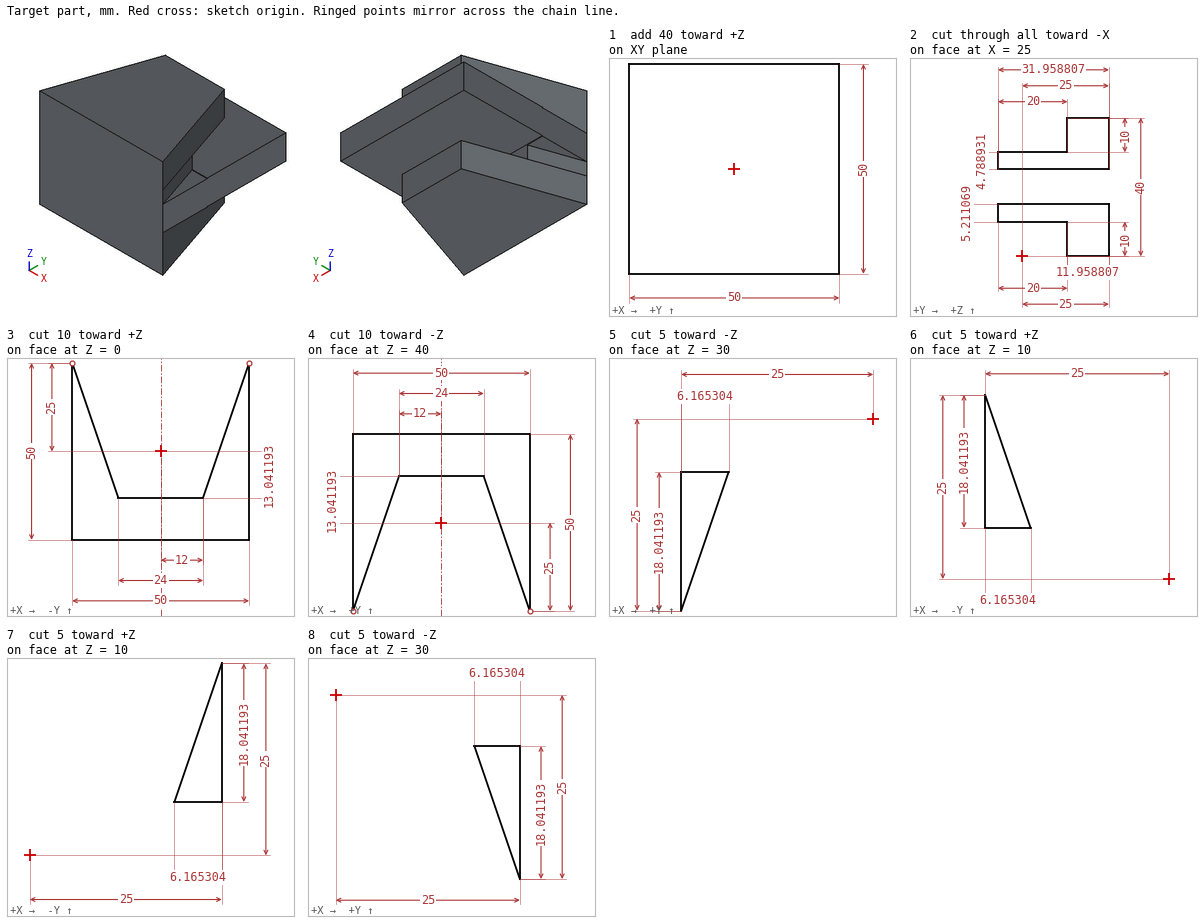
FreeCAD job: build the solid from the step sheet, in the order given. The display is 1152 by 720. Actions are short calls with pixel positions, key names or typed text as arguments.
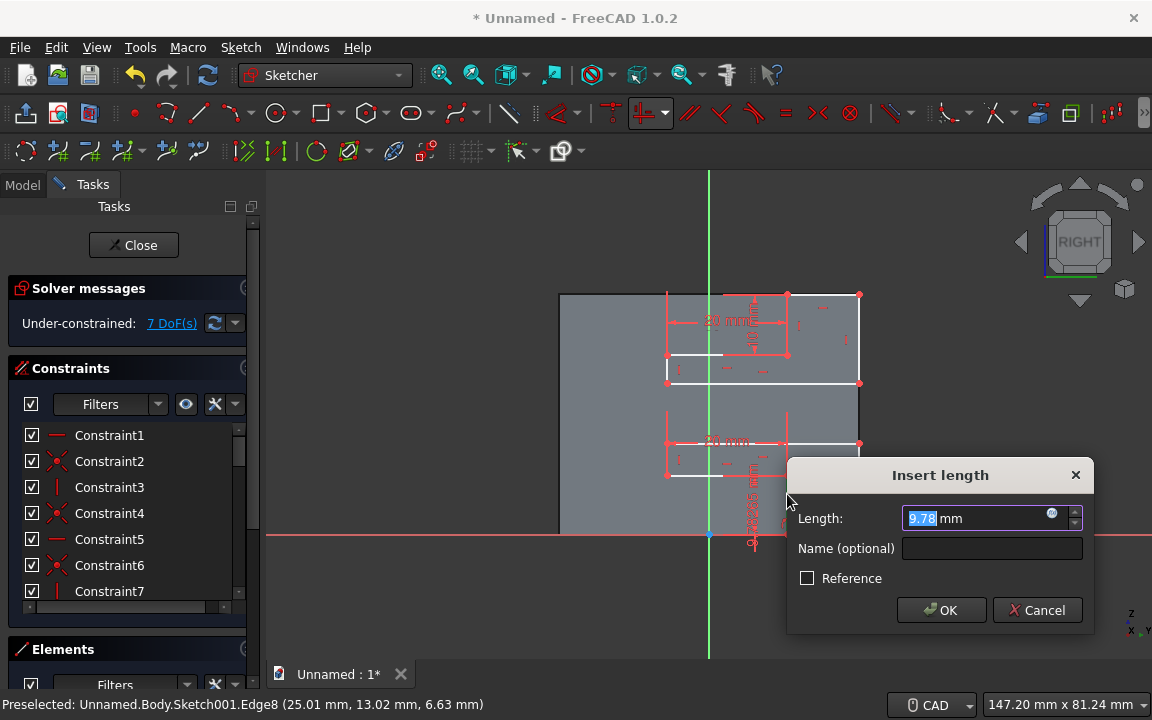
text(10)
key(Return)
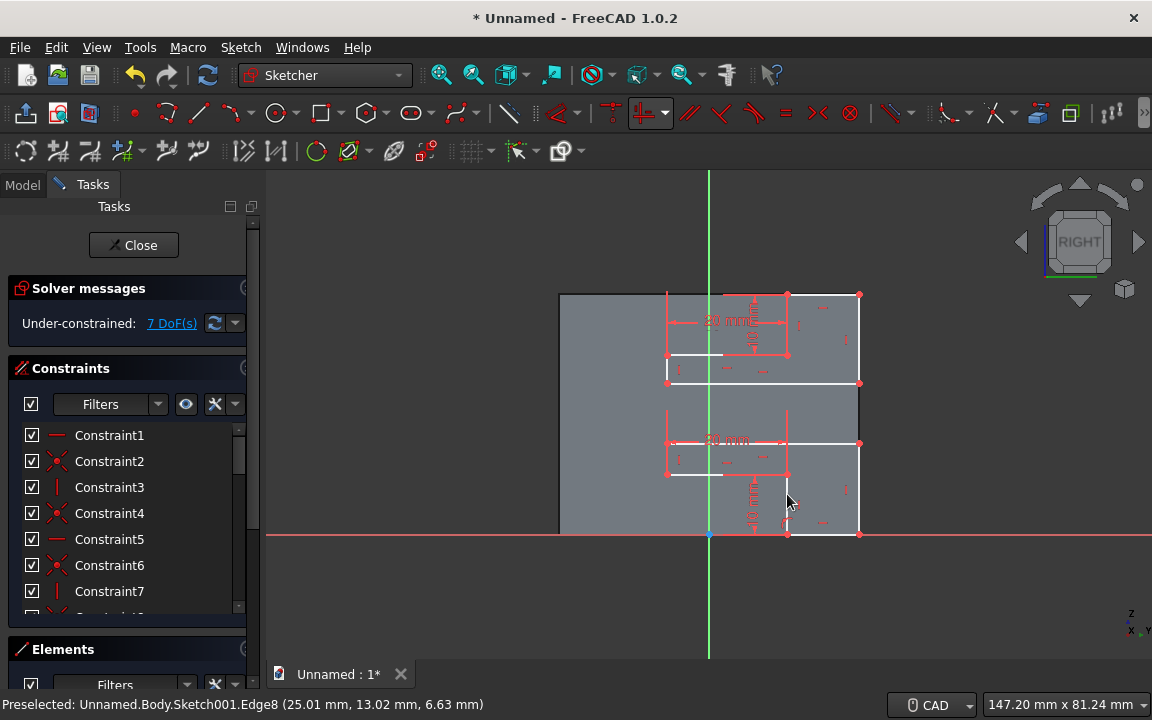
click(859, 384)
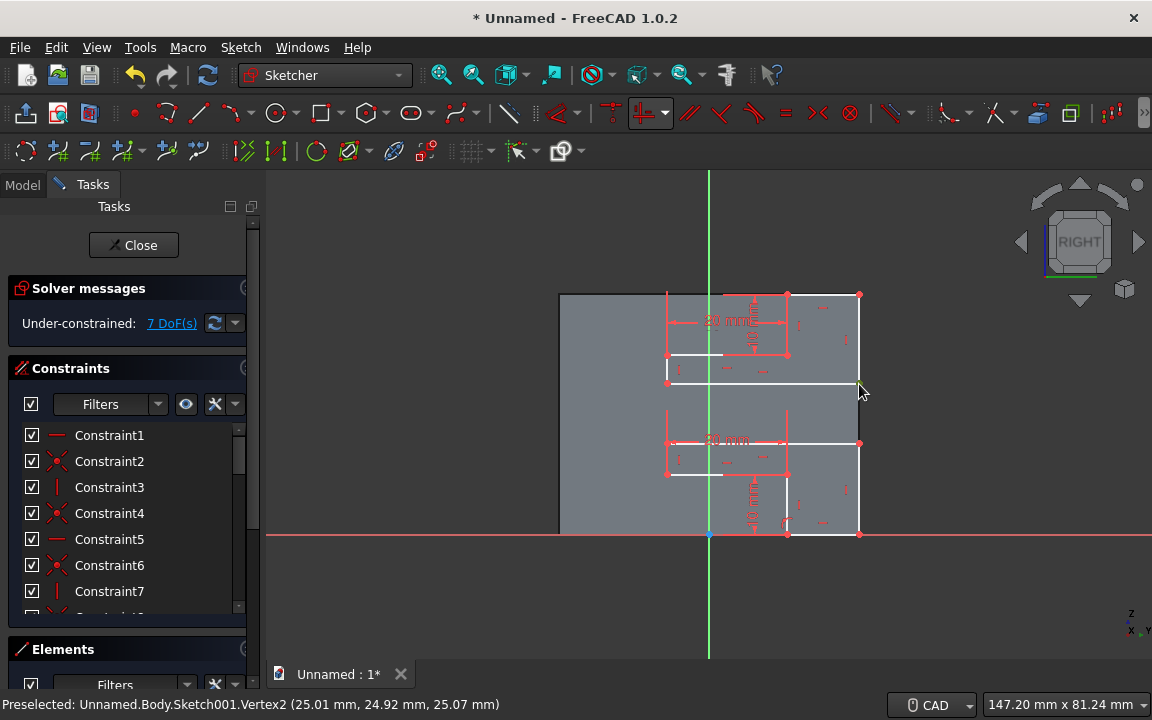
key(l)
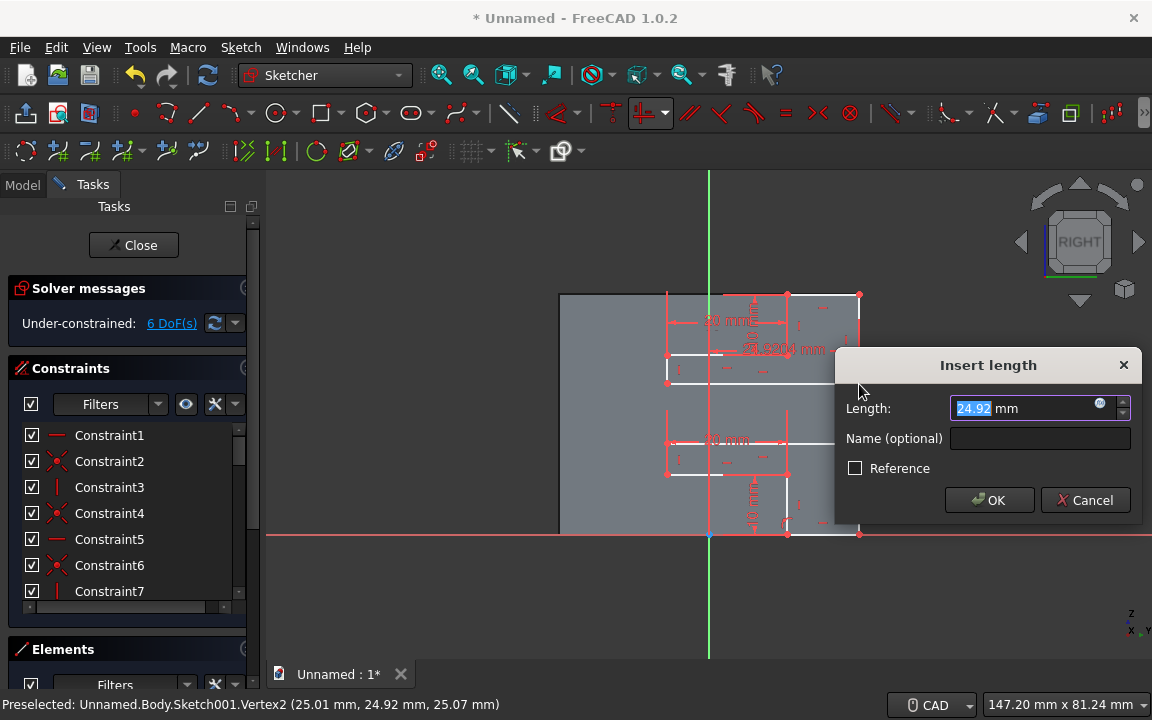
text(25)
key(Return)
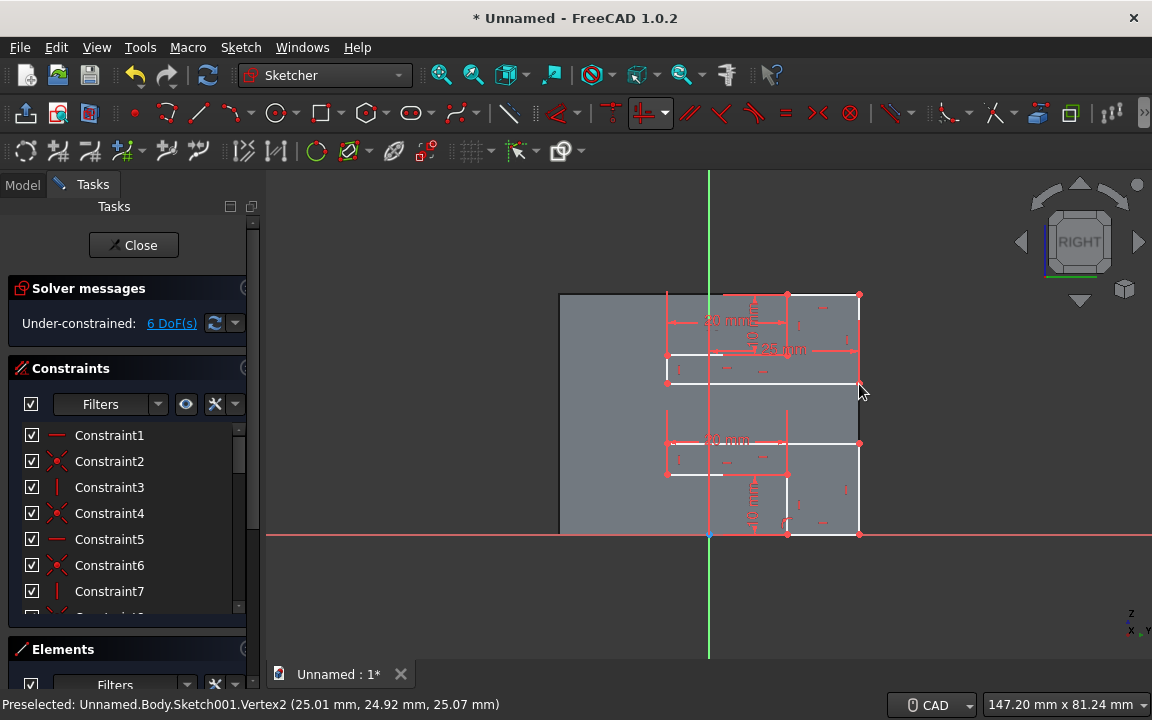
click(859, 295)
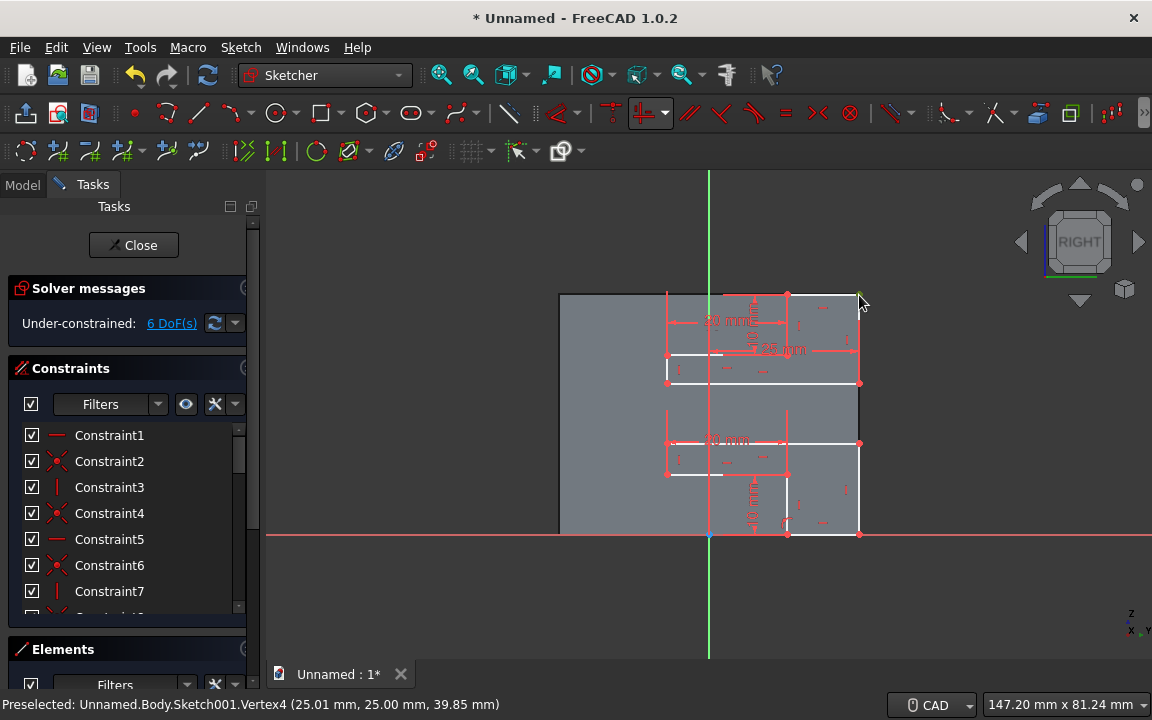
key(i)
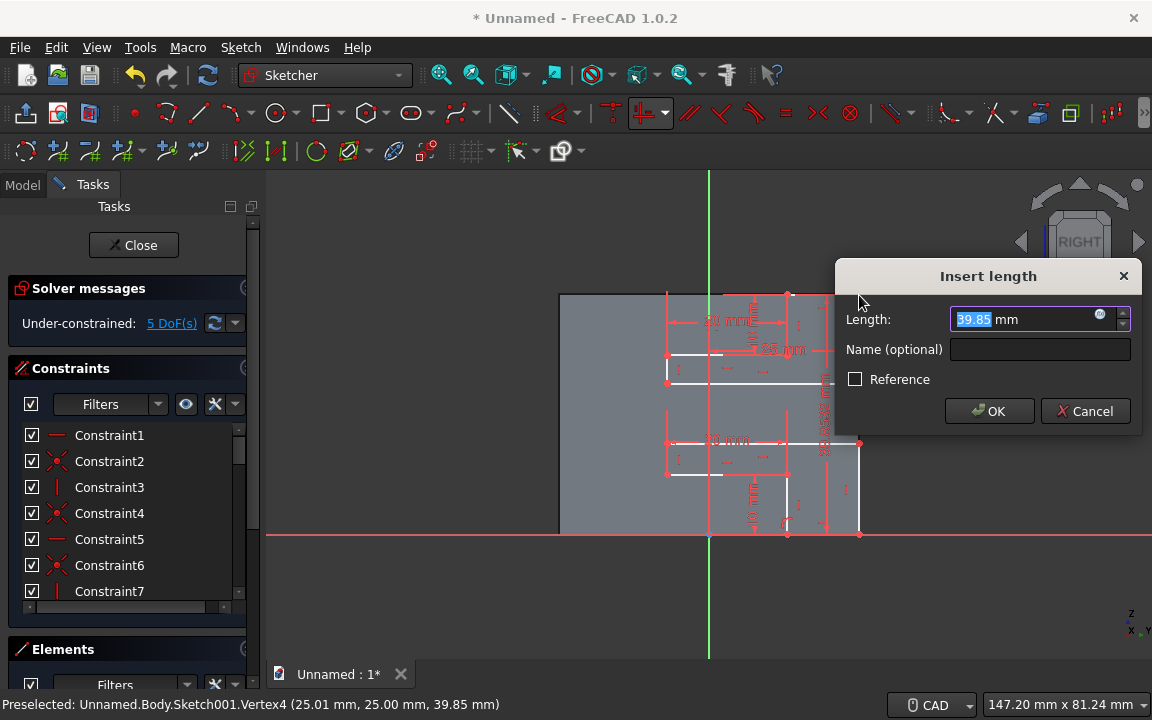
text(40)
key(Return)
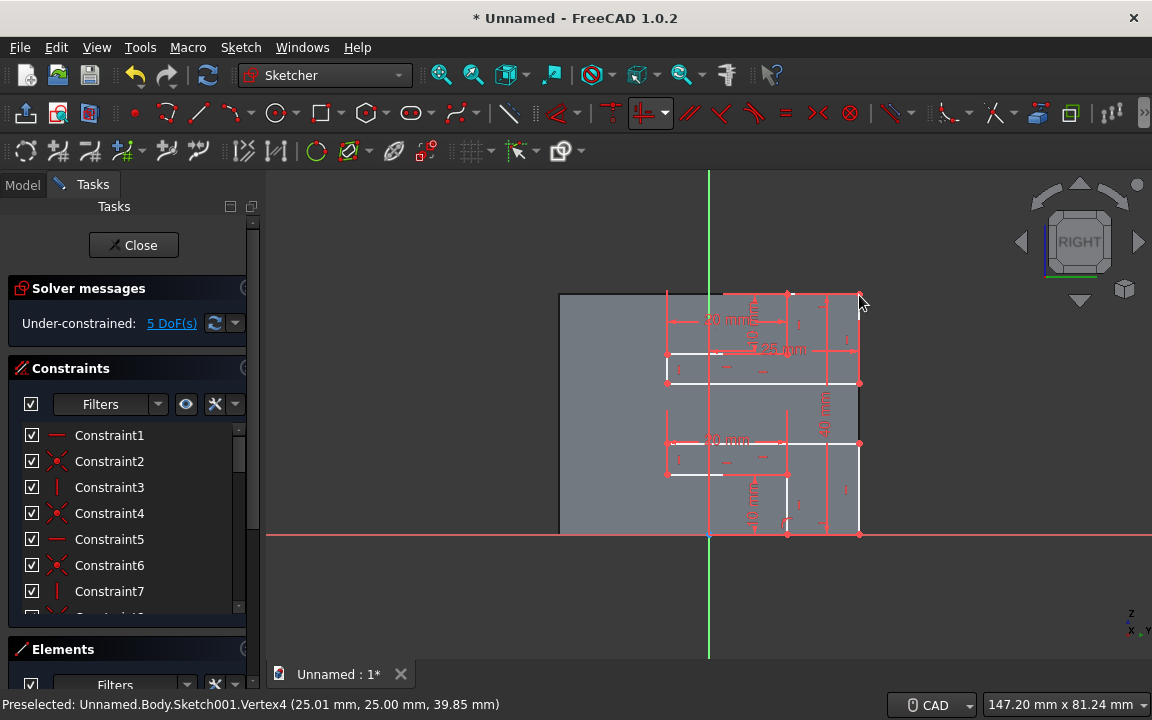
click(859, 535)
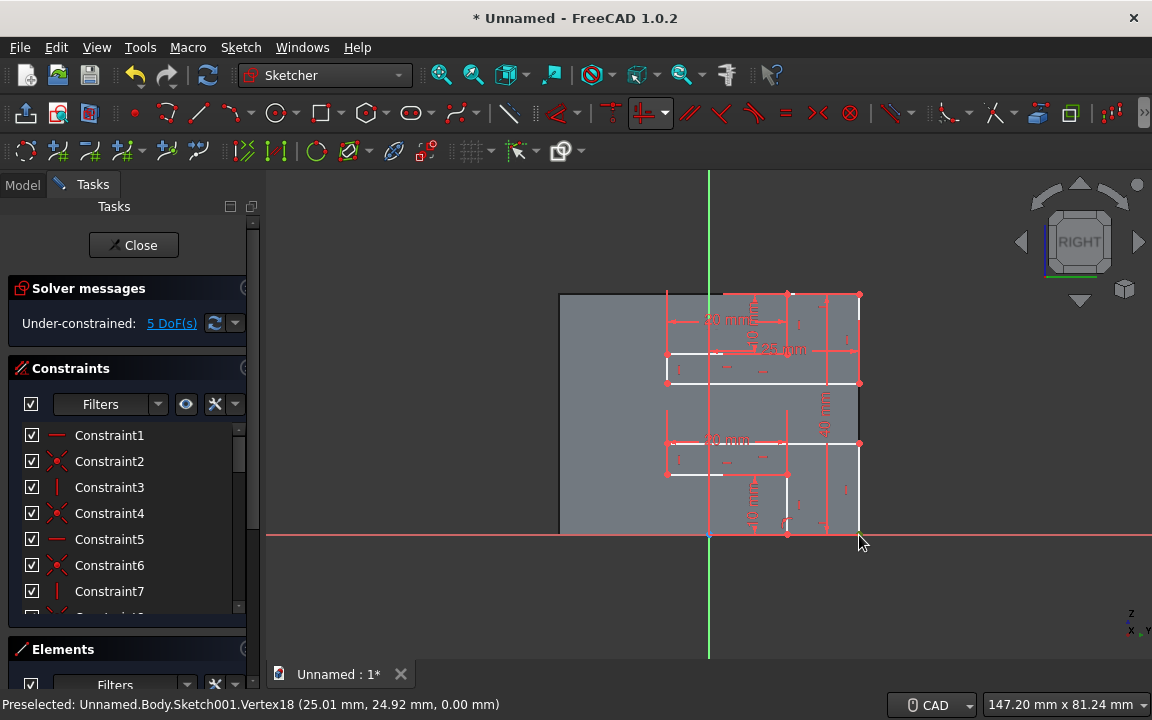
click(580, 114)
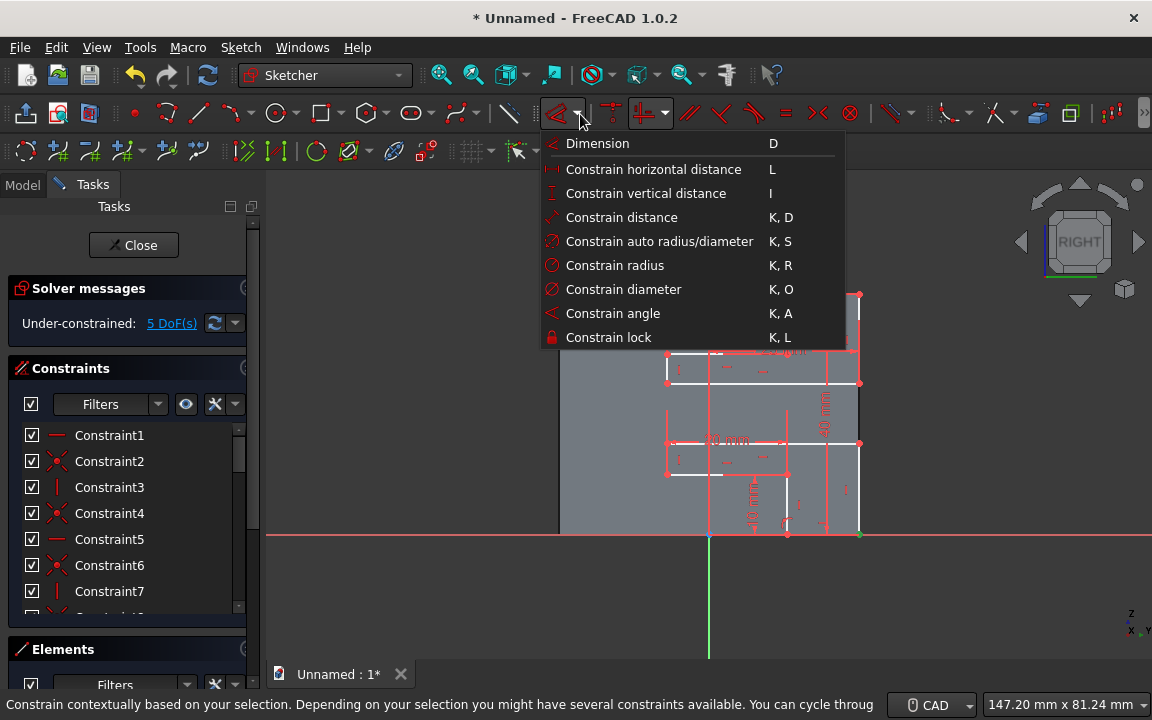
click(693, 169)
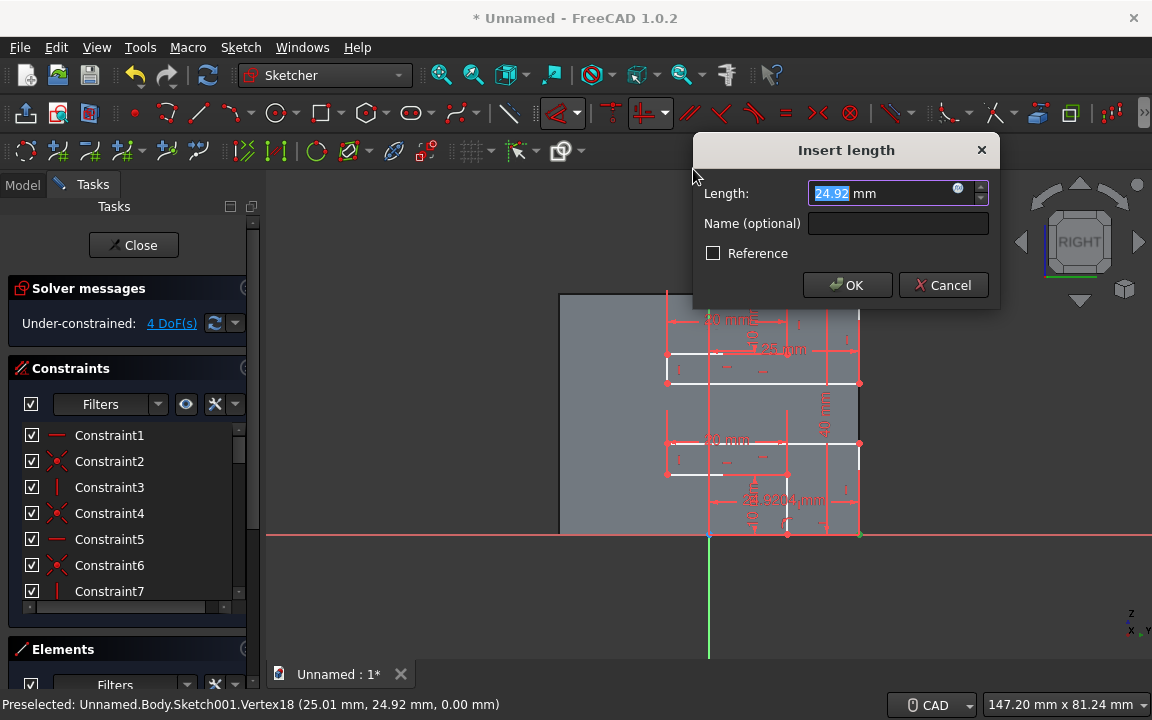
text(25)
key(Return)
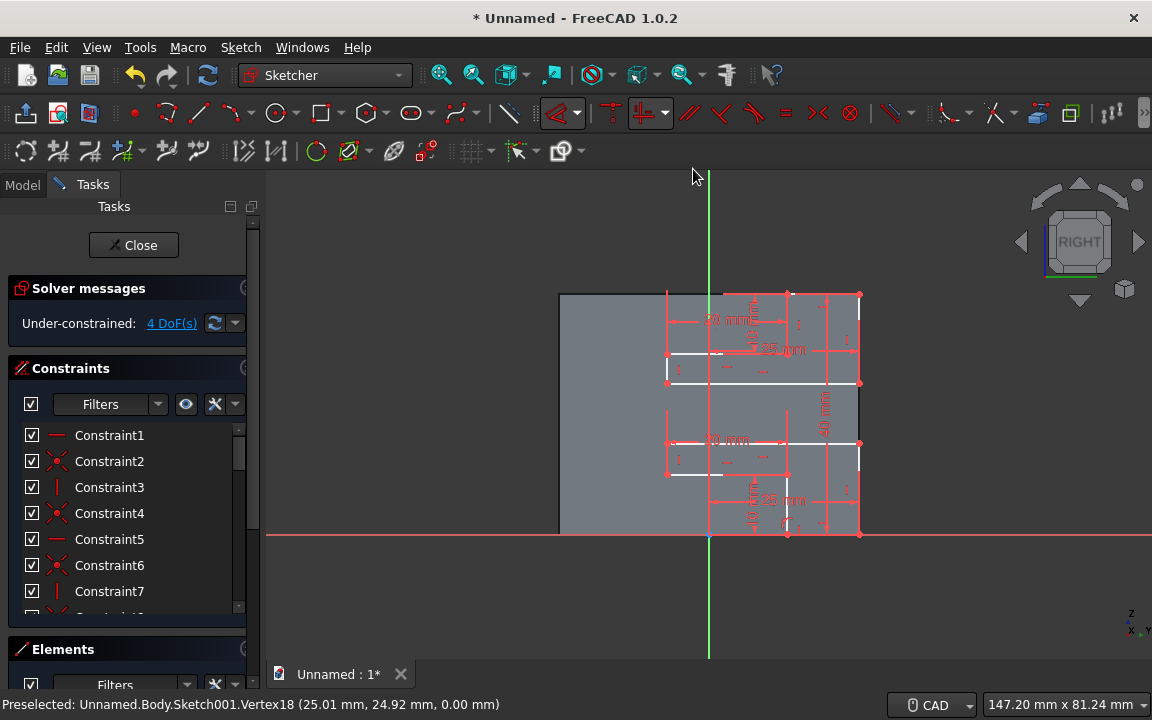
scroll(667, 366, up, 2)